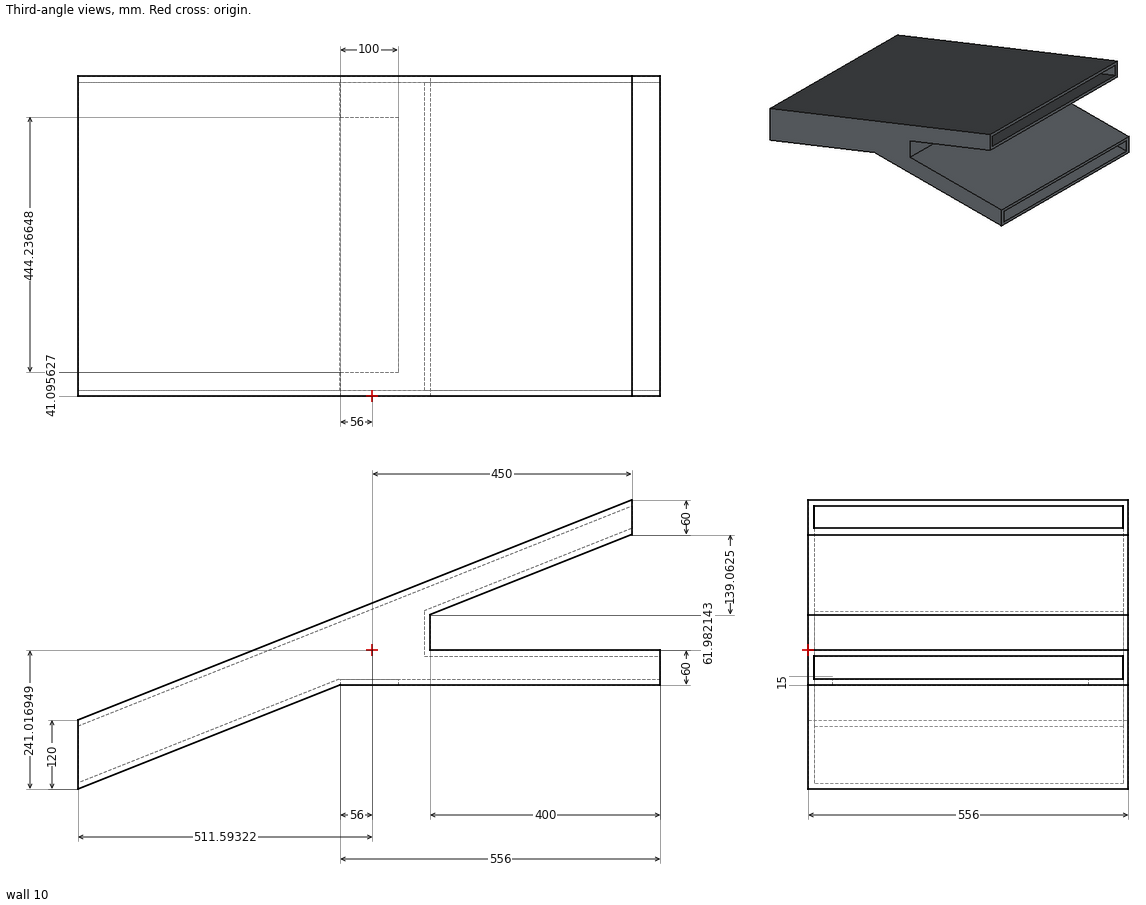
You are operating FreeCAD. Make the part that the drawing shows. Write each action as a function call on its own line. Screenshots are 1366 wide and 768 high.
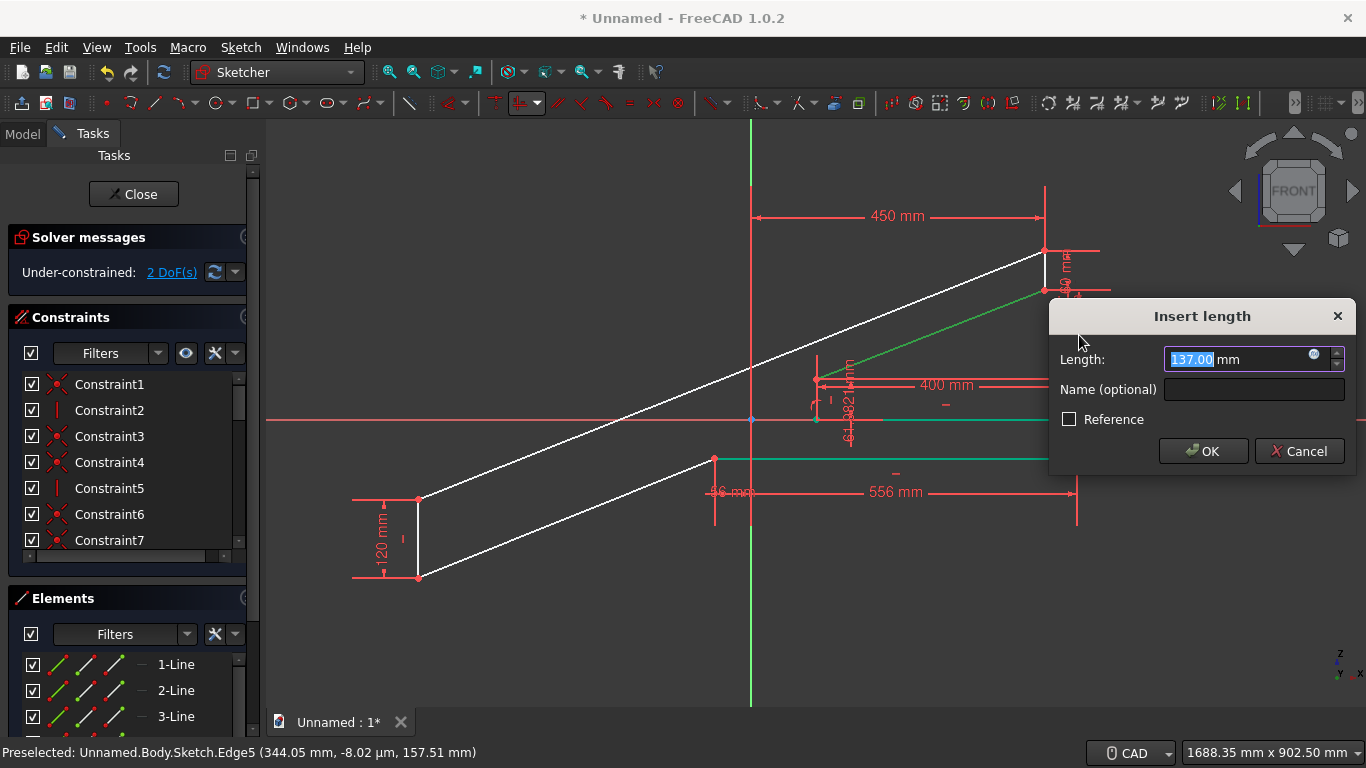
text(139.0625)
key(Return)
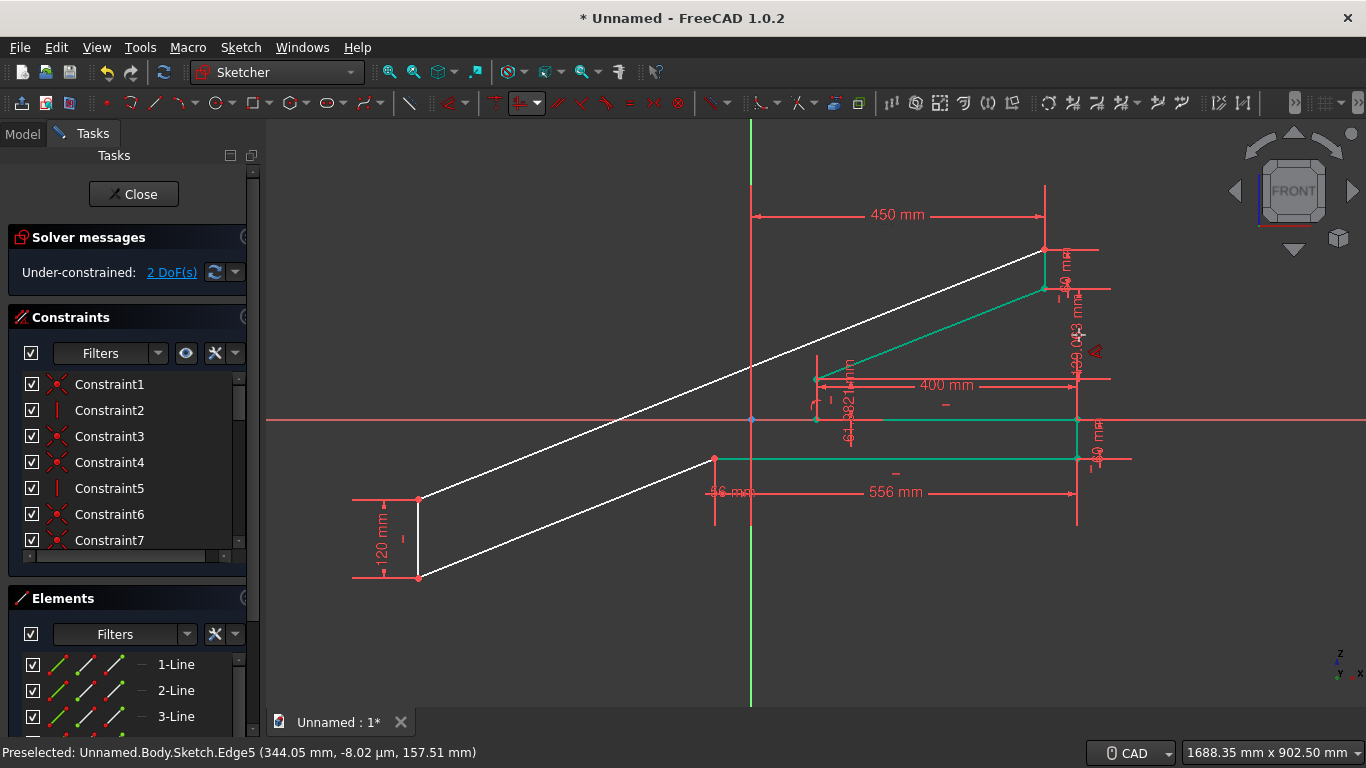
click(418, 578)
click(585, 612)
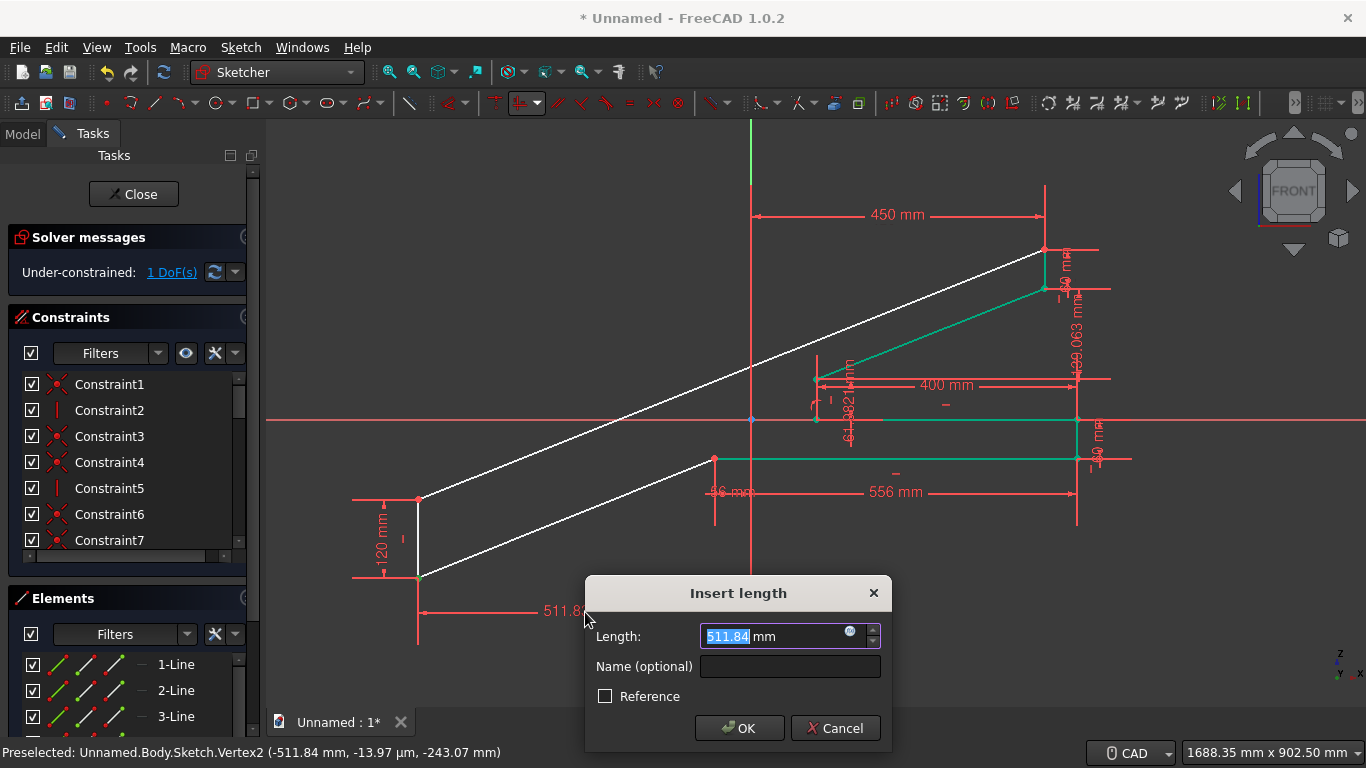
text(511.59322)
key(Return)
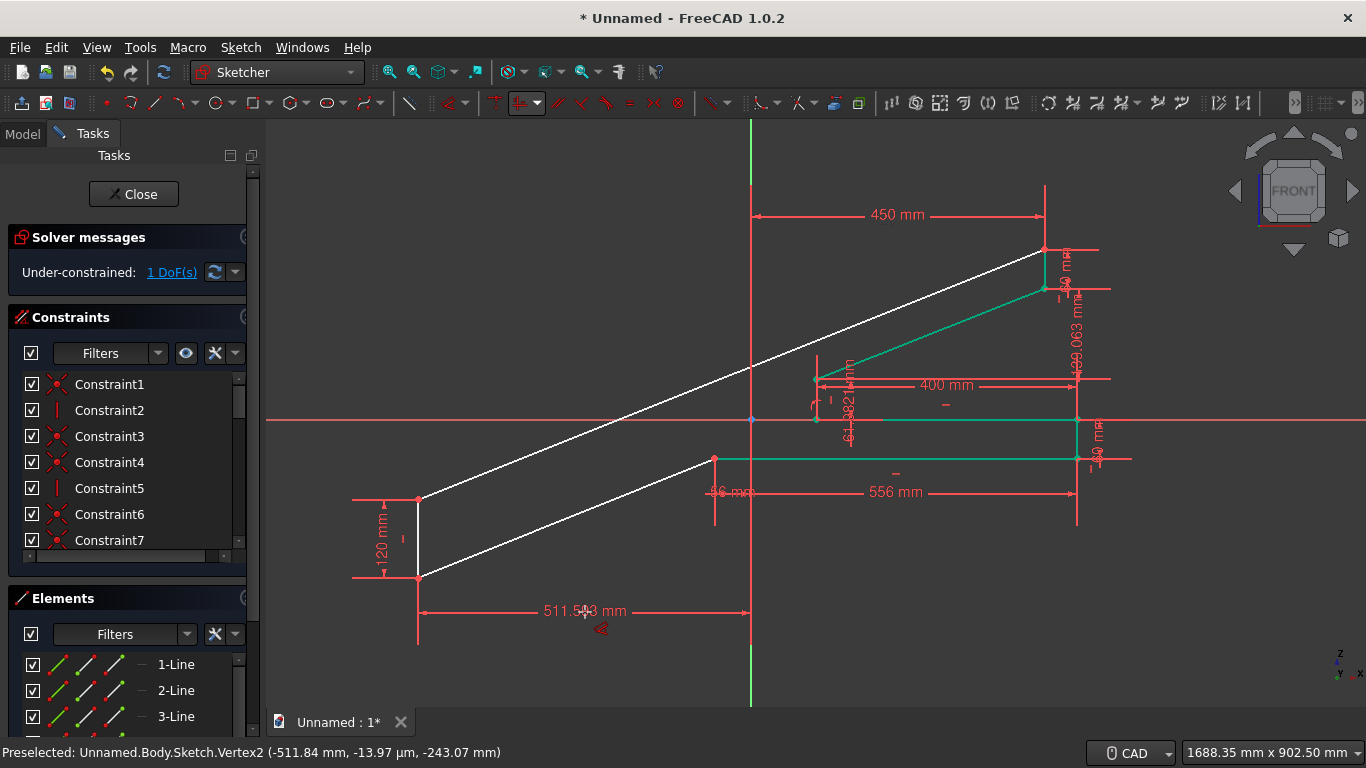
click(418, 578)
click(384, 499)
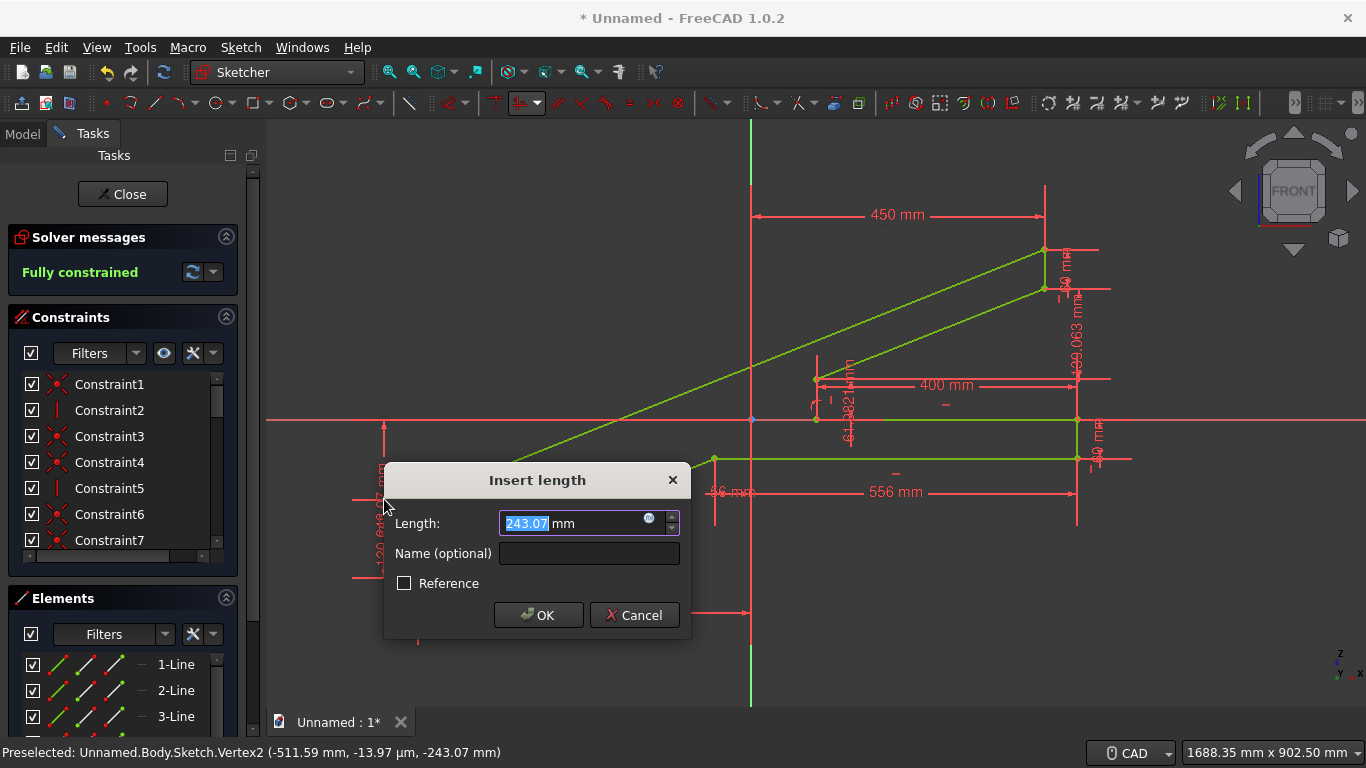
text(241.016949)
key(Return)
key(Escape)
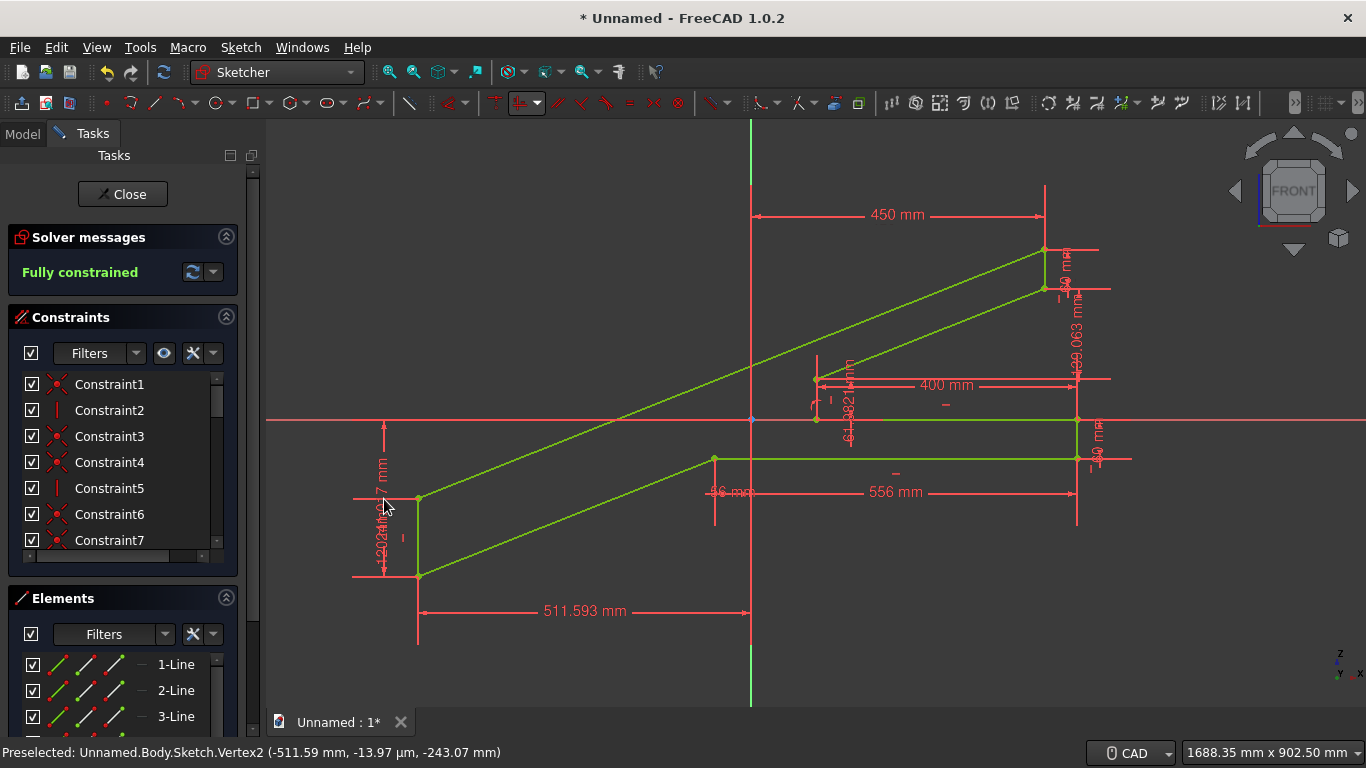
click(123, 194)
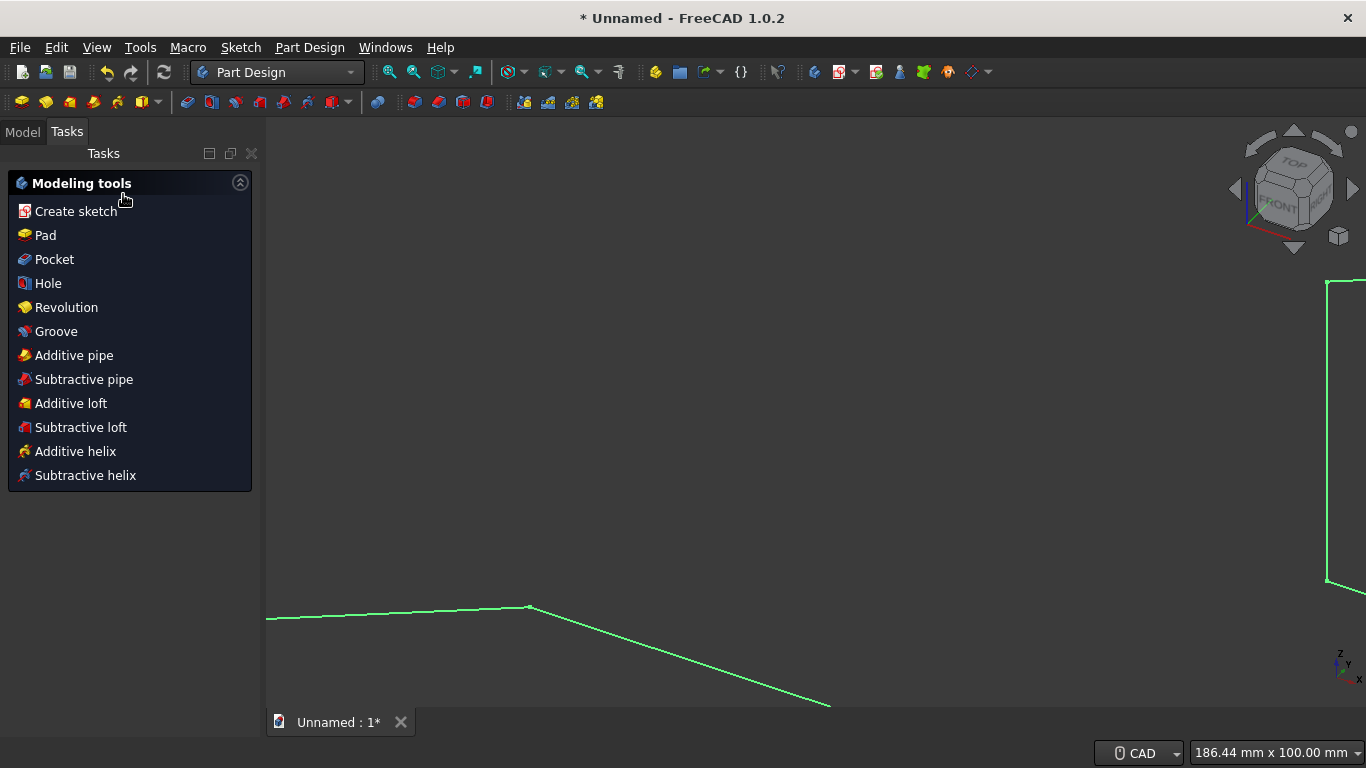
click(22, 102)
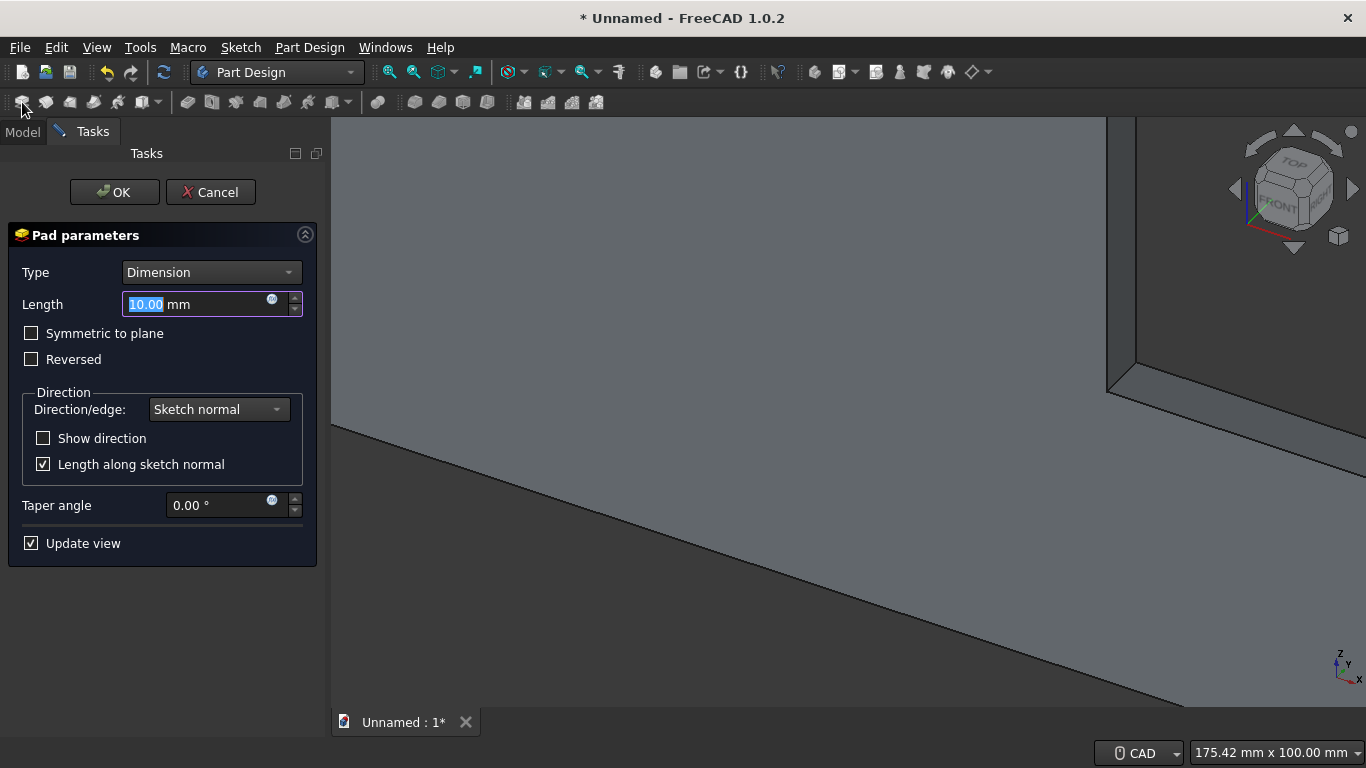
text(556)
key(Tab)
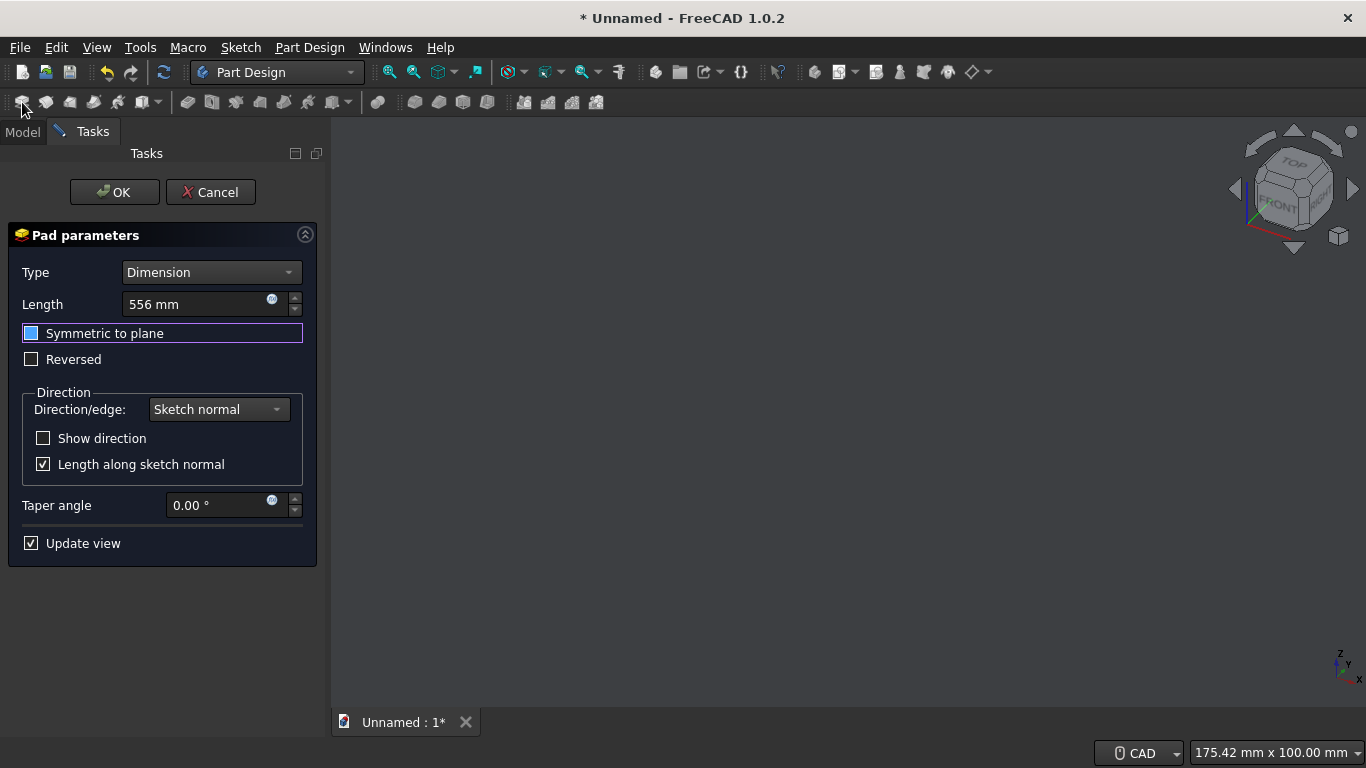
click(30, 359)